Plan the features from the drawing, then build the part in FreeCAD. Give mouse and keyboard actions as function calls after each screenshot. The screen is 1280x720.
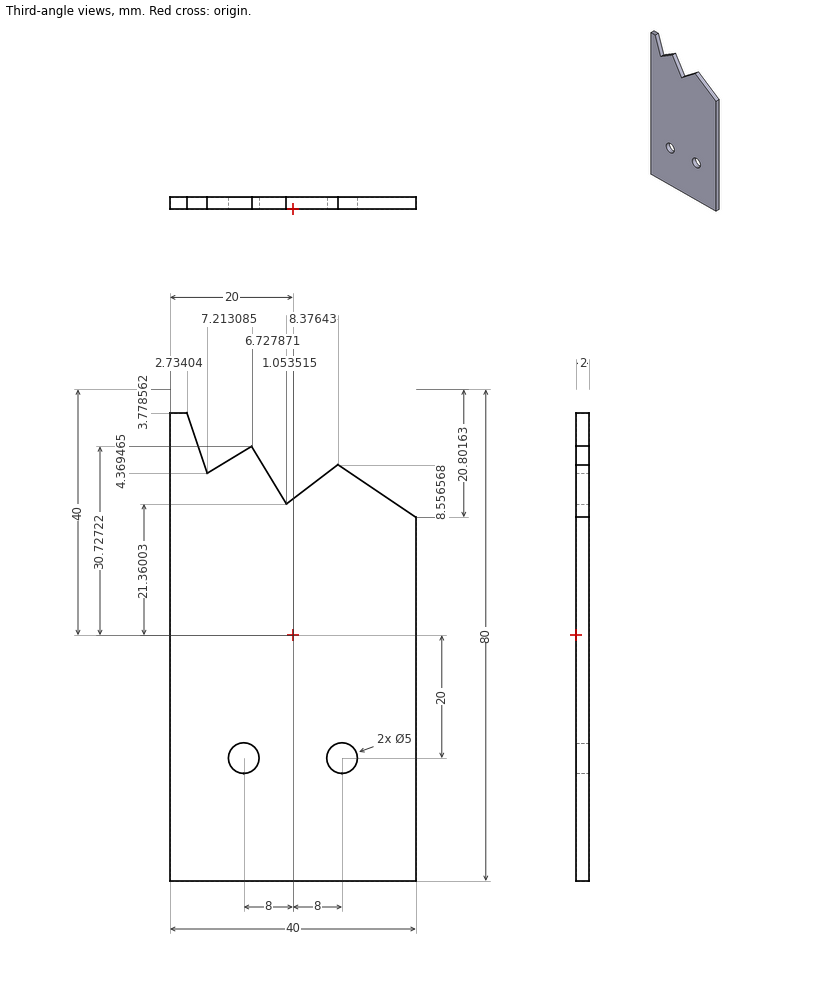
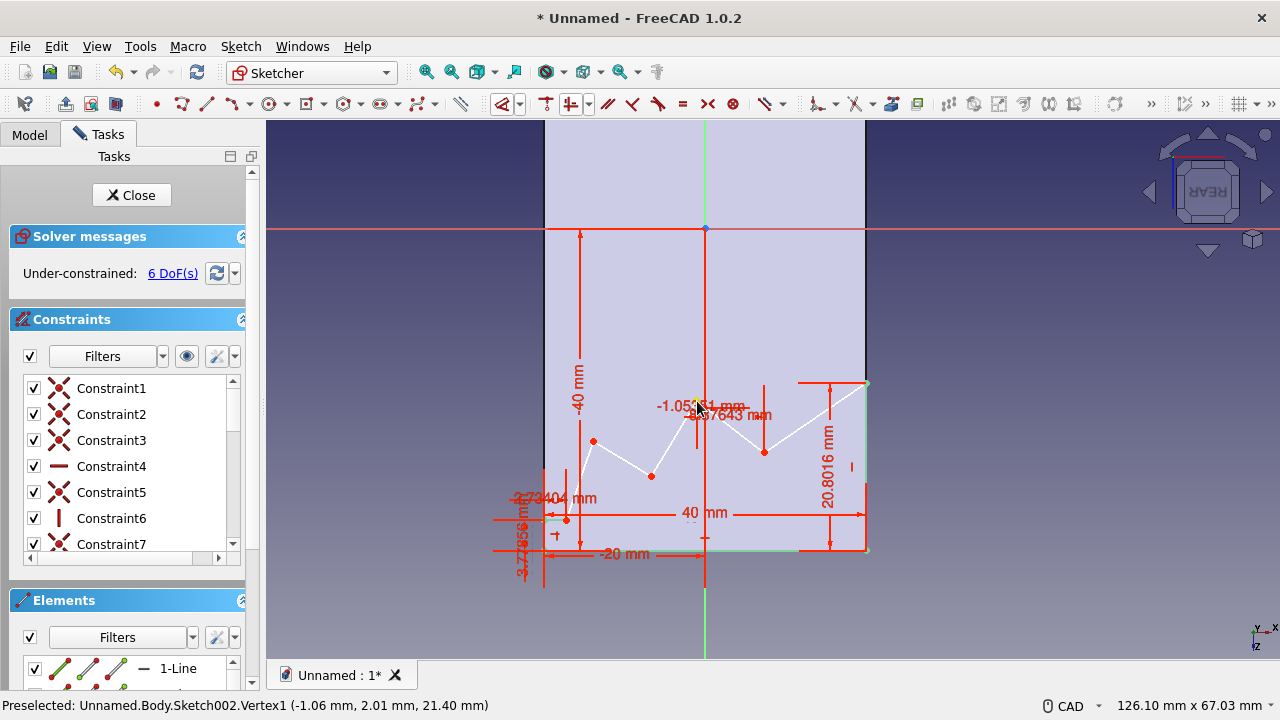
click(697, 401)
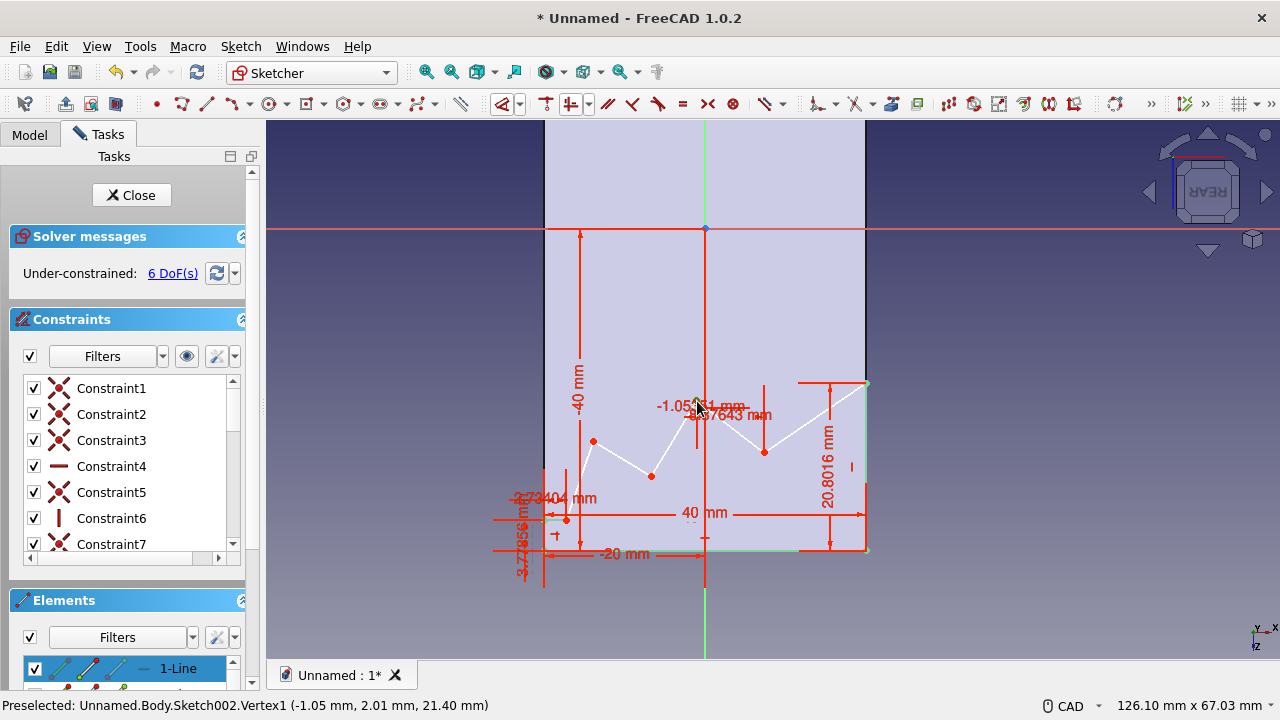
key(i)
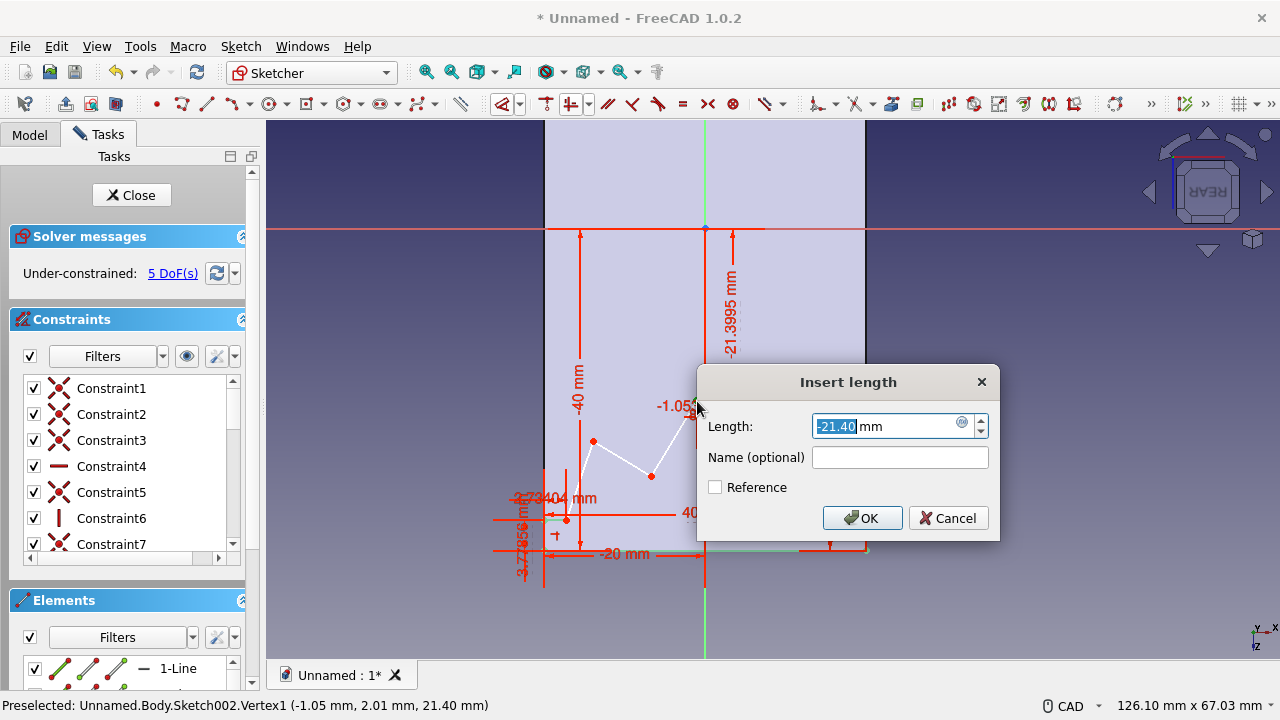
text(-21.36003)
key(Return)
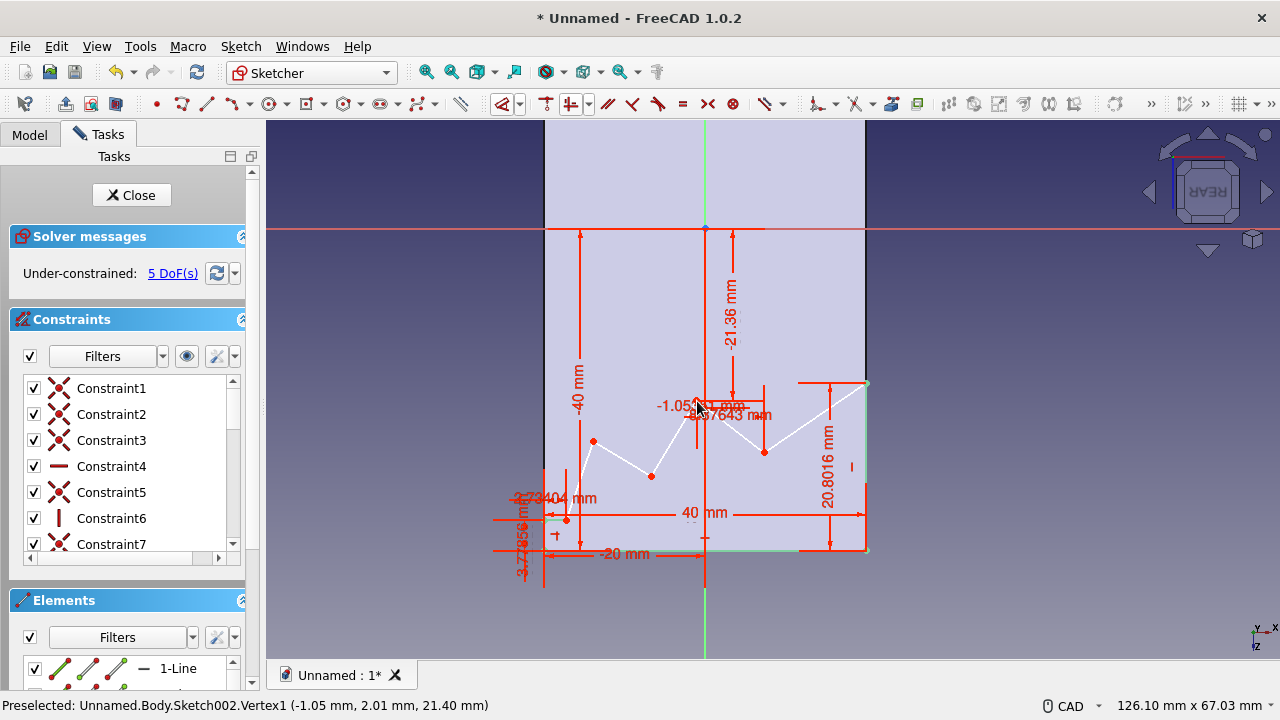
click(651, 476)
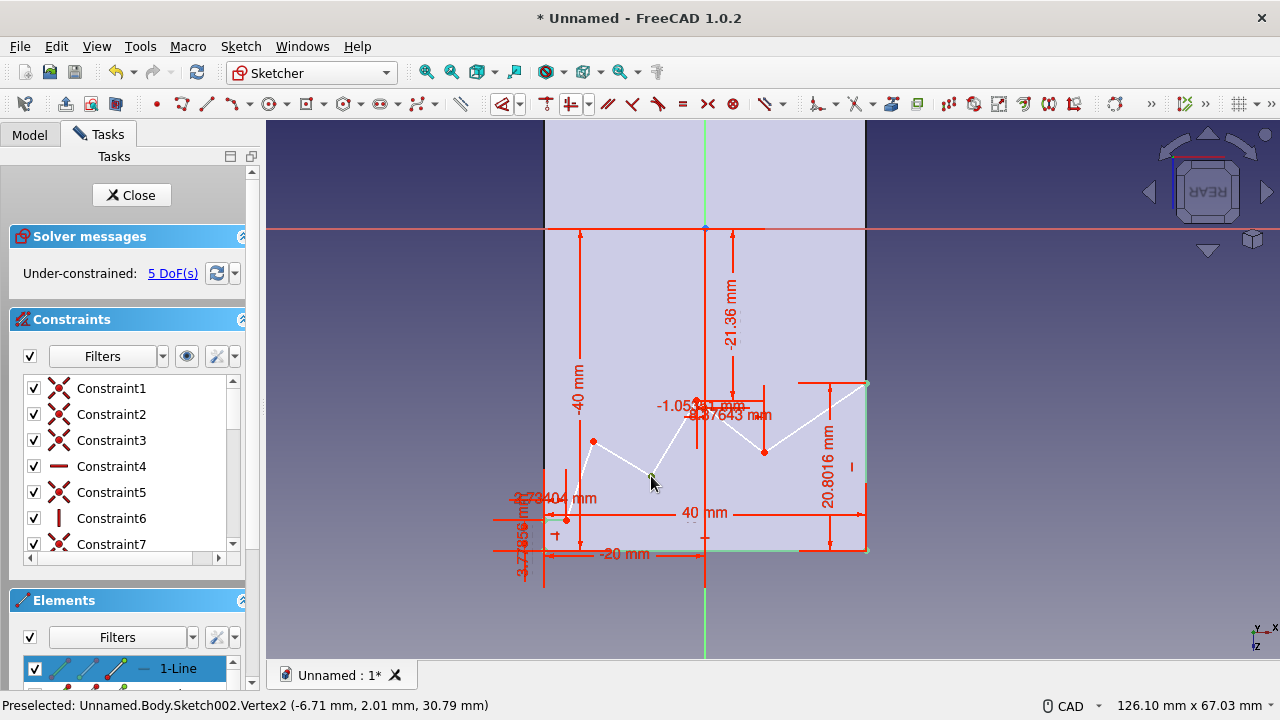
key(l)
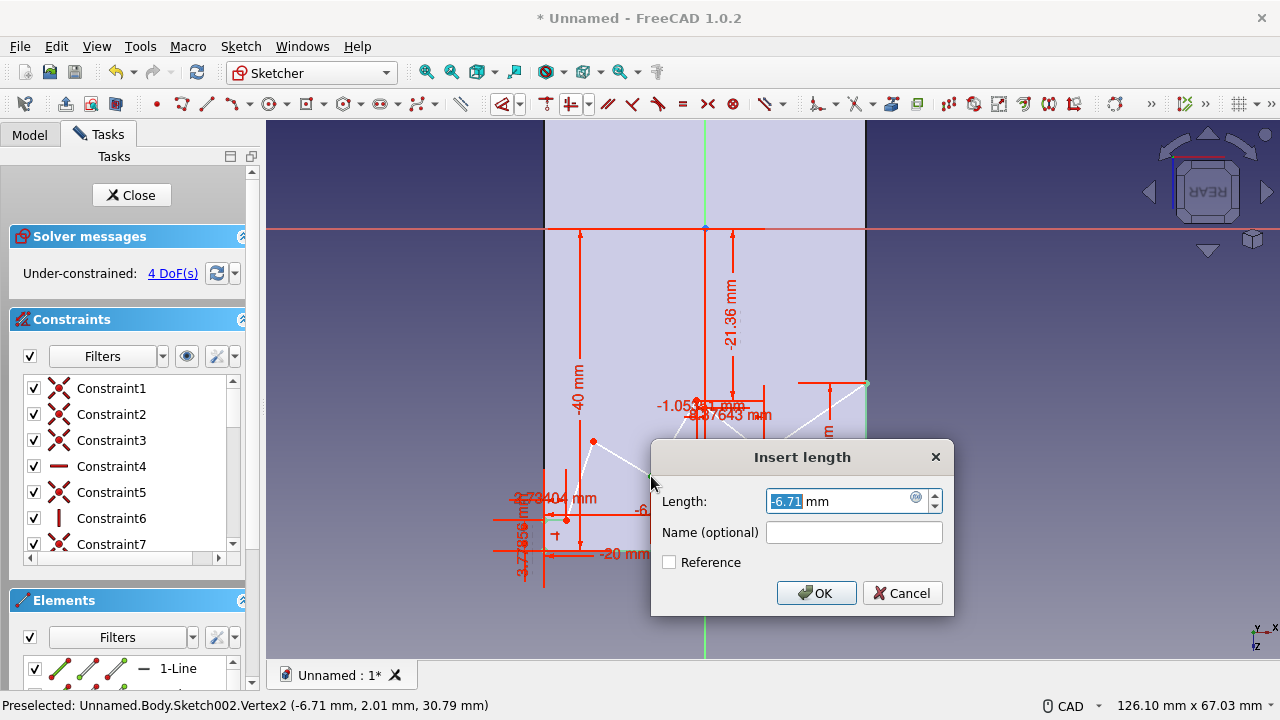
text(-6.727871)
key(Return)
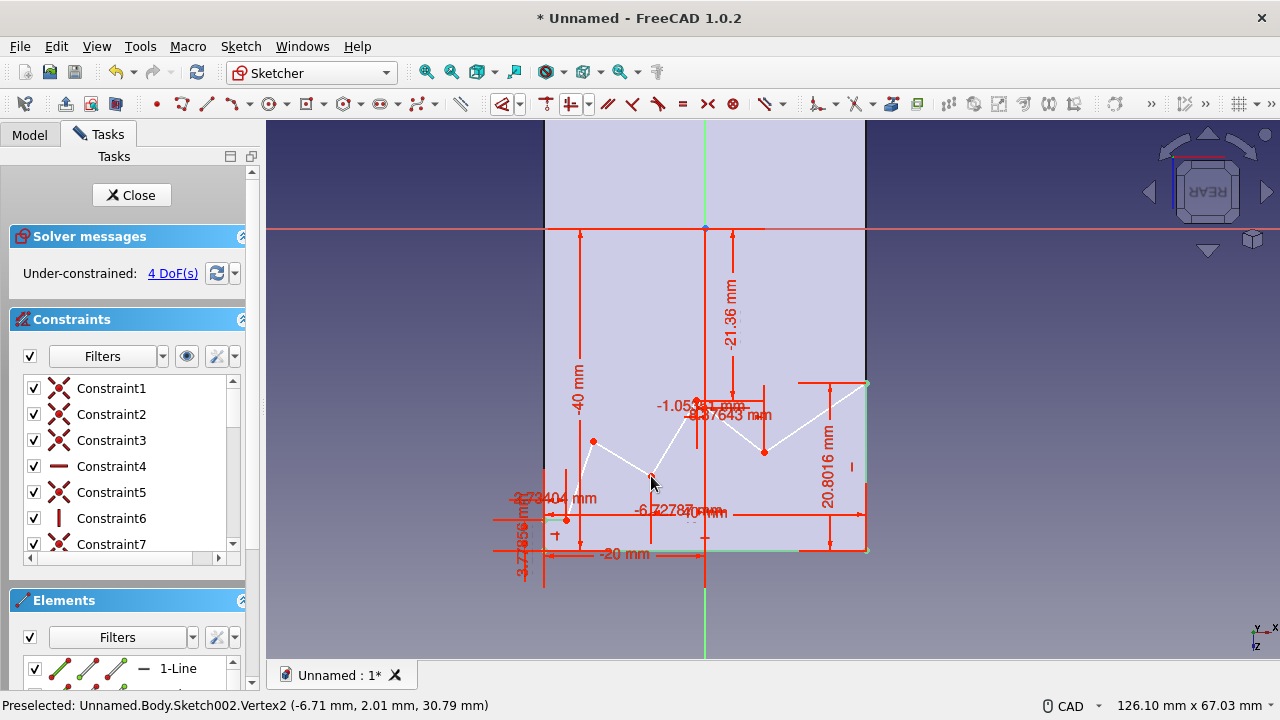
click(651, 476)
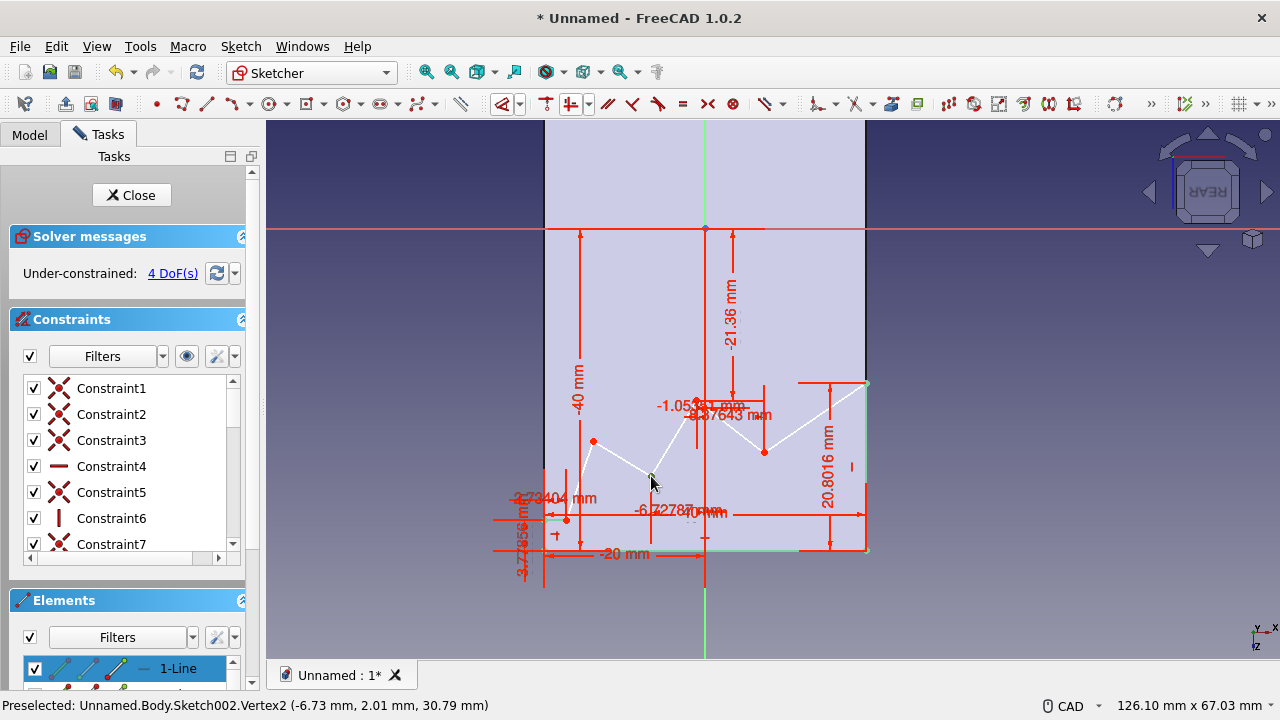
key(i)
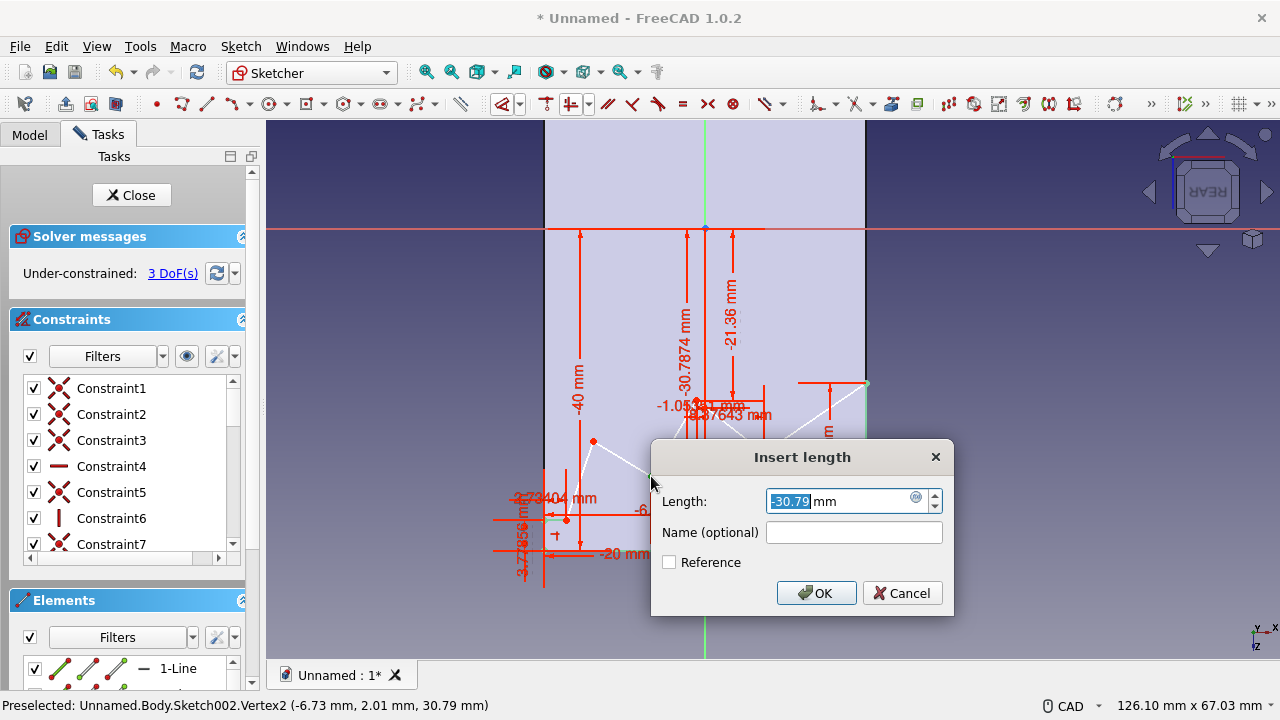
text(-30.72722)
key(Return)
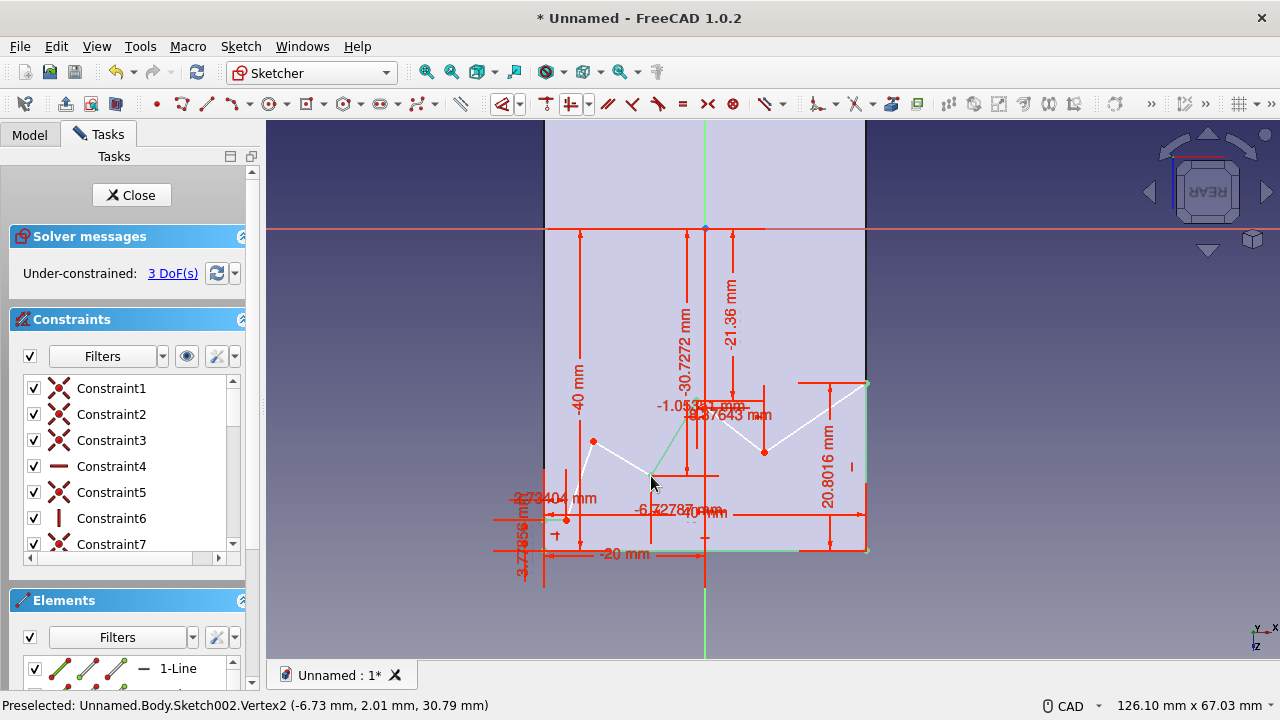
click(634, 466)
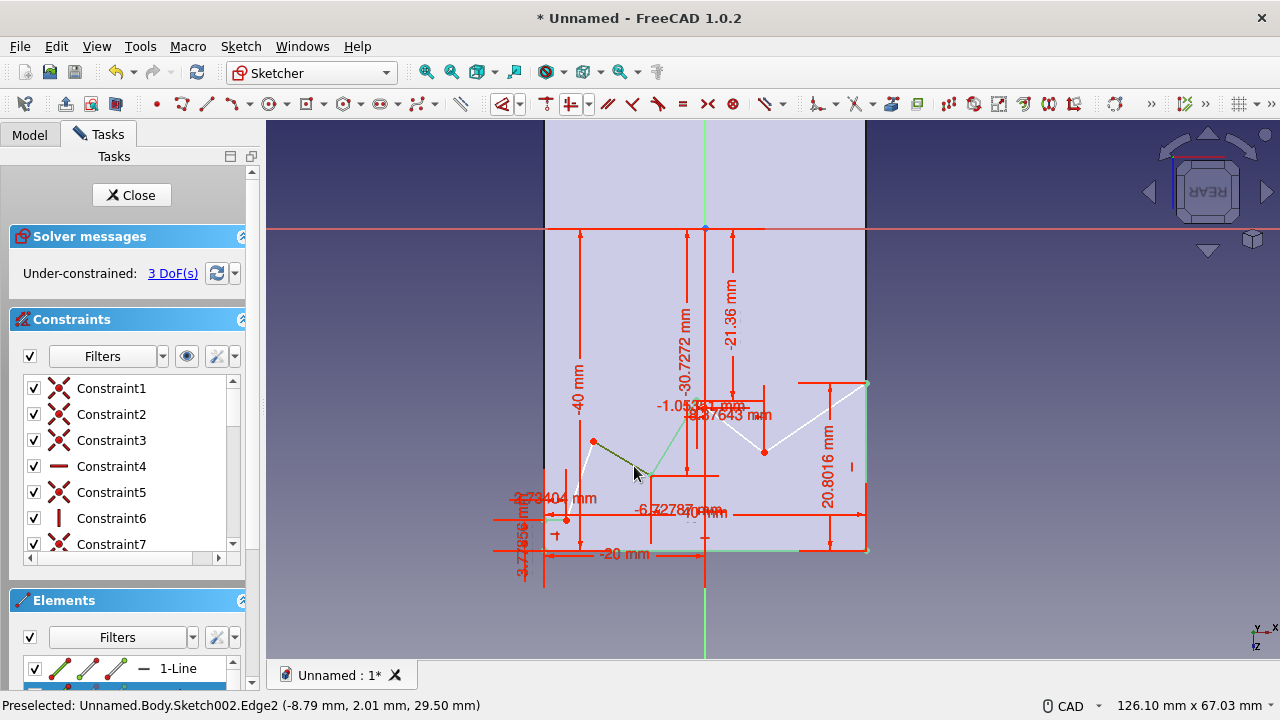
key(l)